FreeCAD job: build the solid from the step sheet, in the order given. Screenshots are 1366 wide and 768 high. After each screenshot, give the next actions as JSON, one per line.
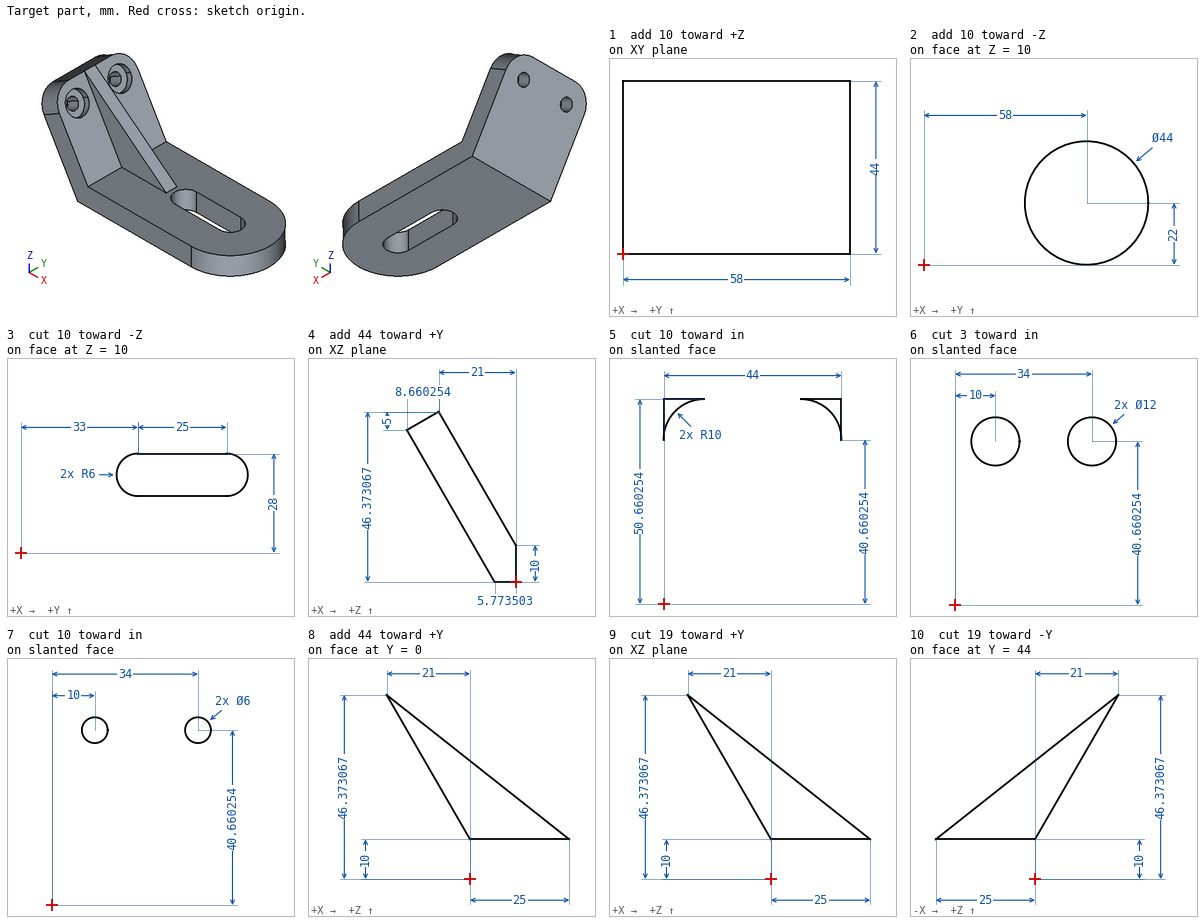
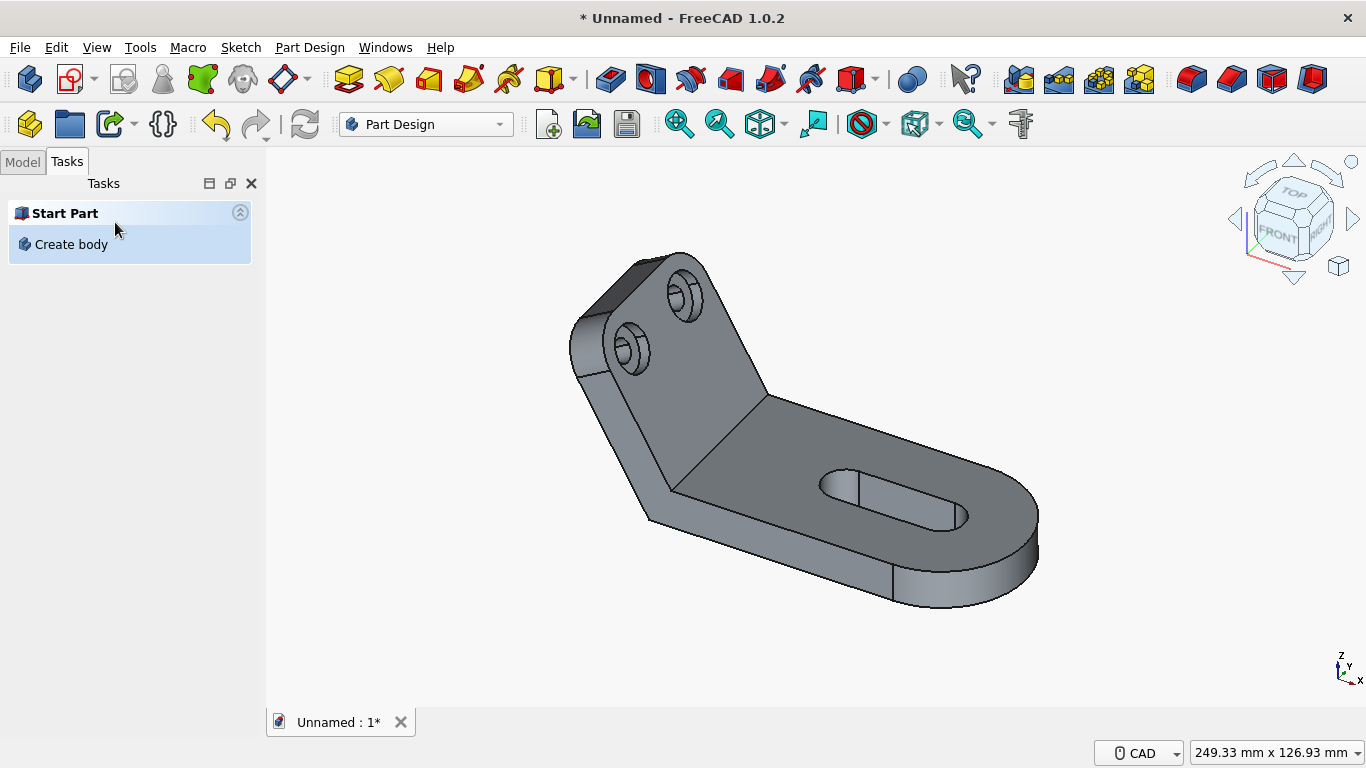
{"action": "left_click", "coordinate": [645, 469]}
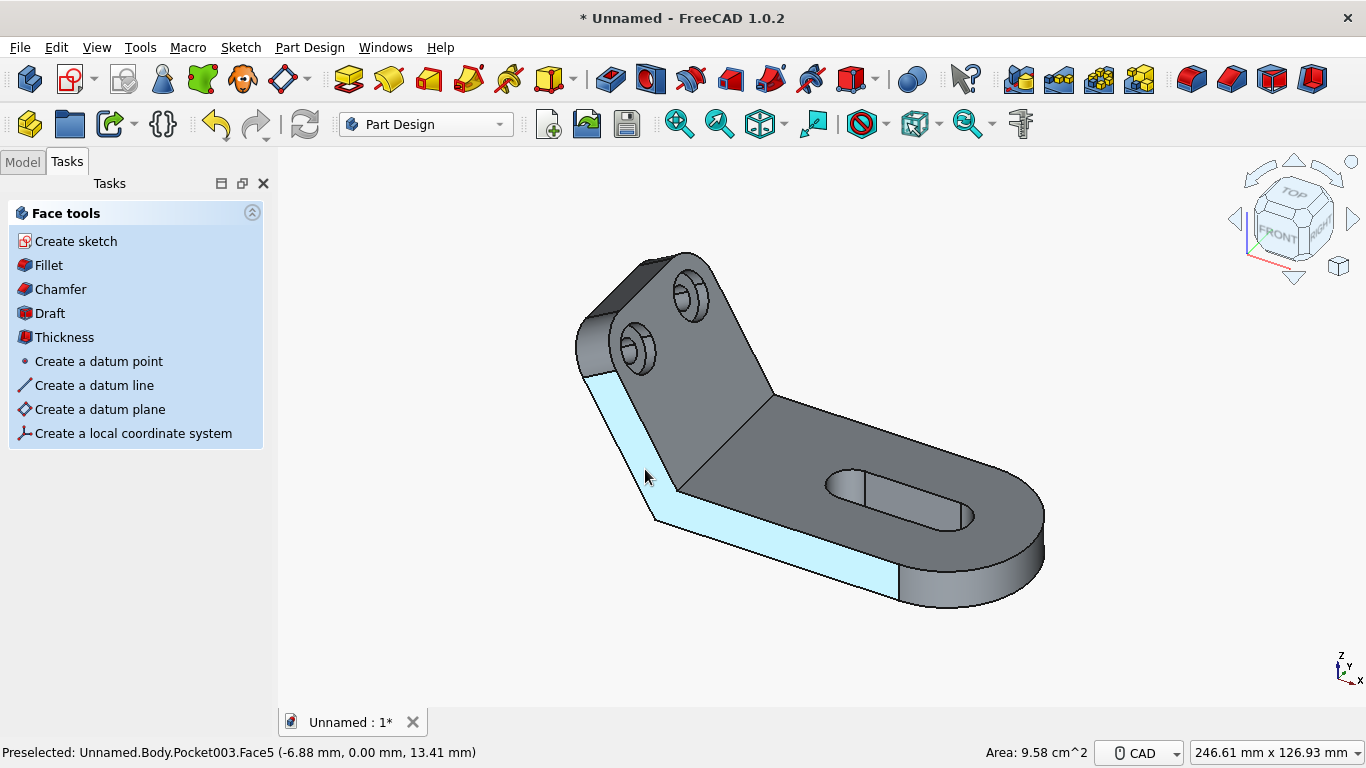
{"action": "left_click", "coordinate": [70, 80]}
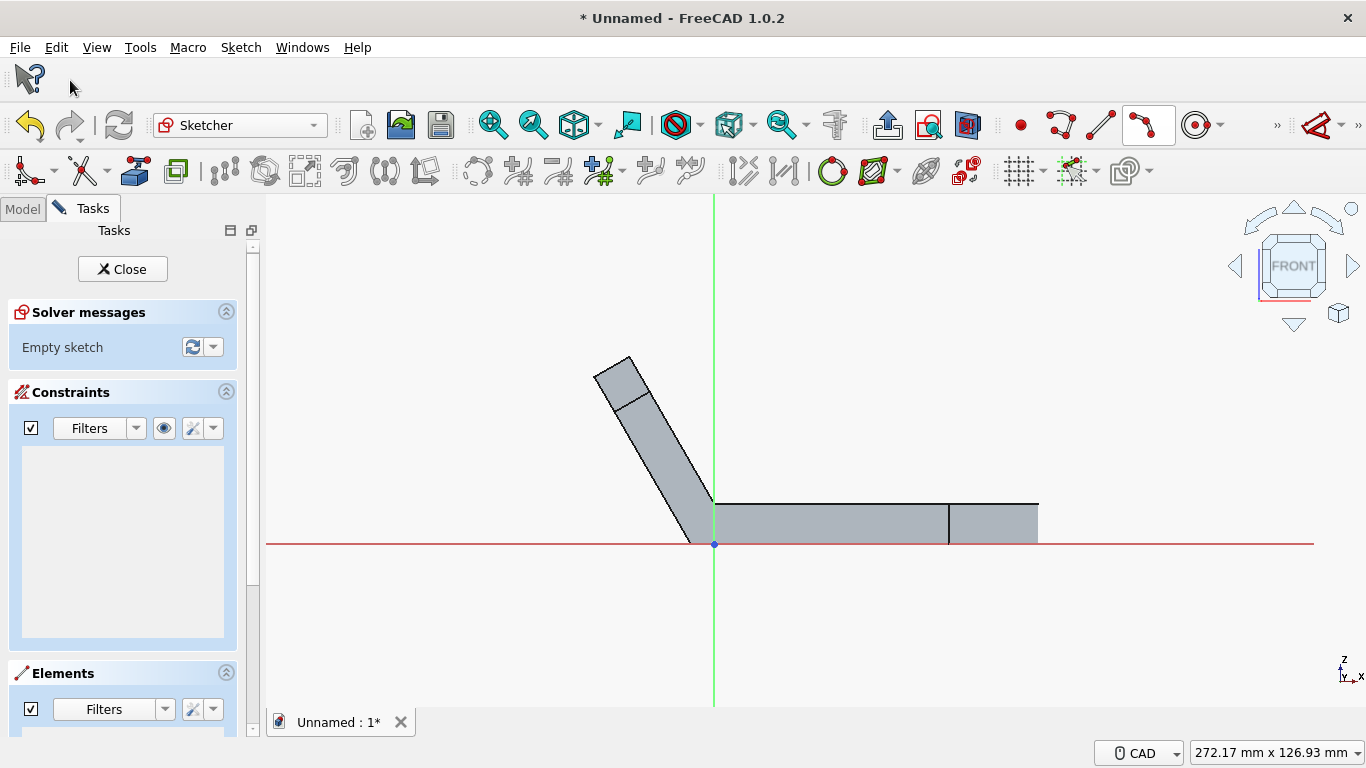
{"action": "scroll", "coordinate": [692, 451], "scroll_direction": "up", "scroll_amount": 3}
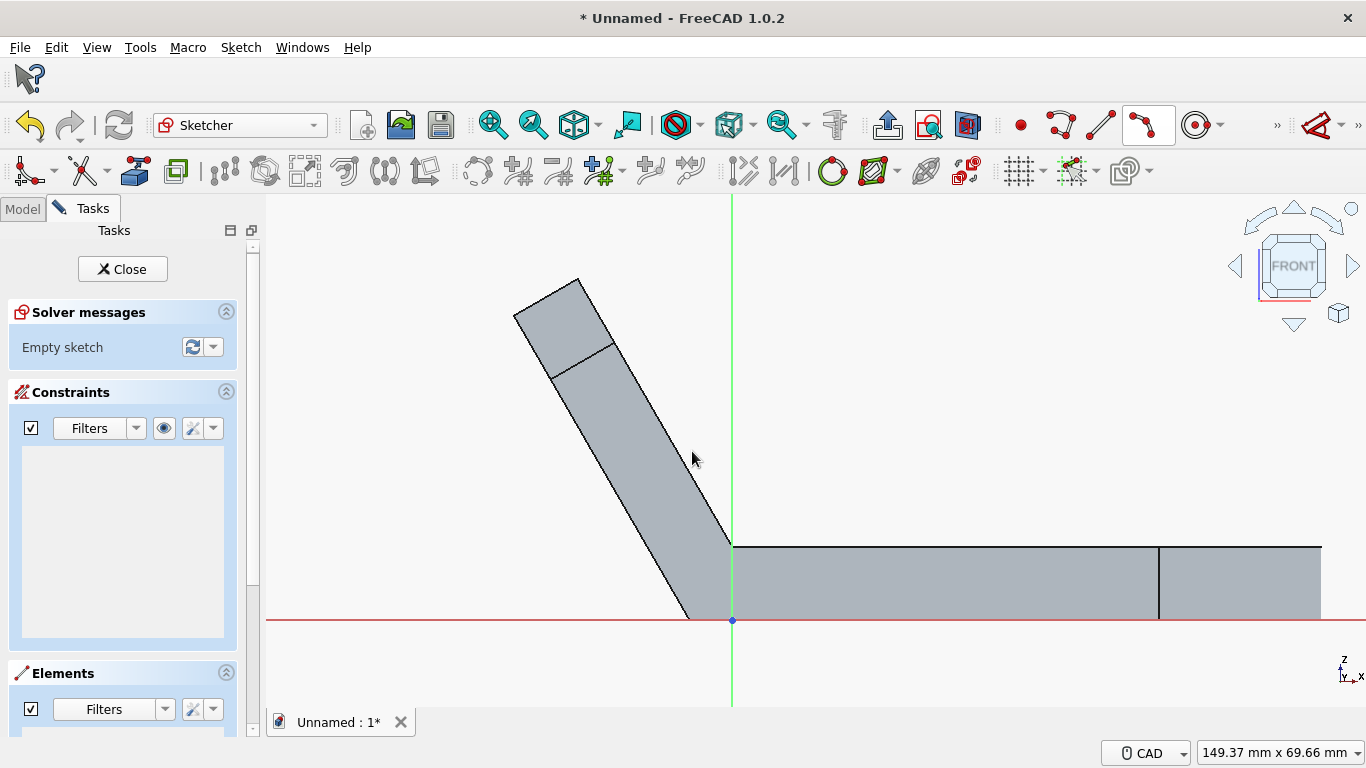
{"action": "left_click", "coordinate": [1062, 126]}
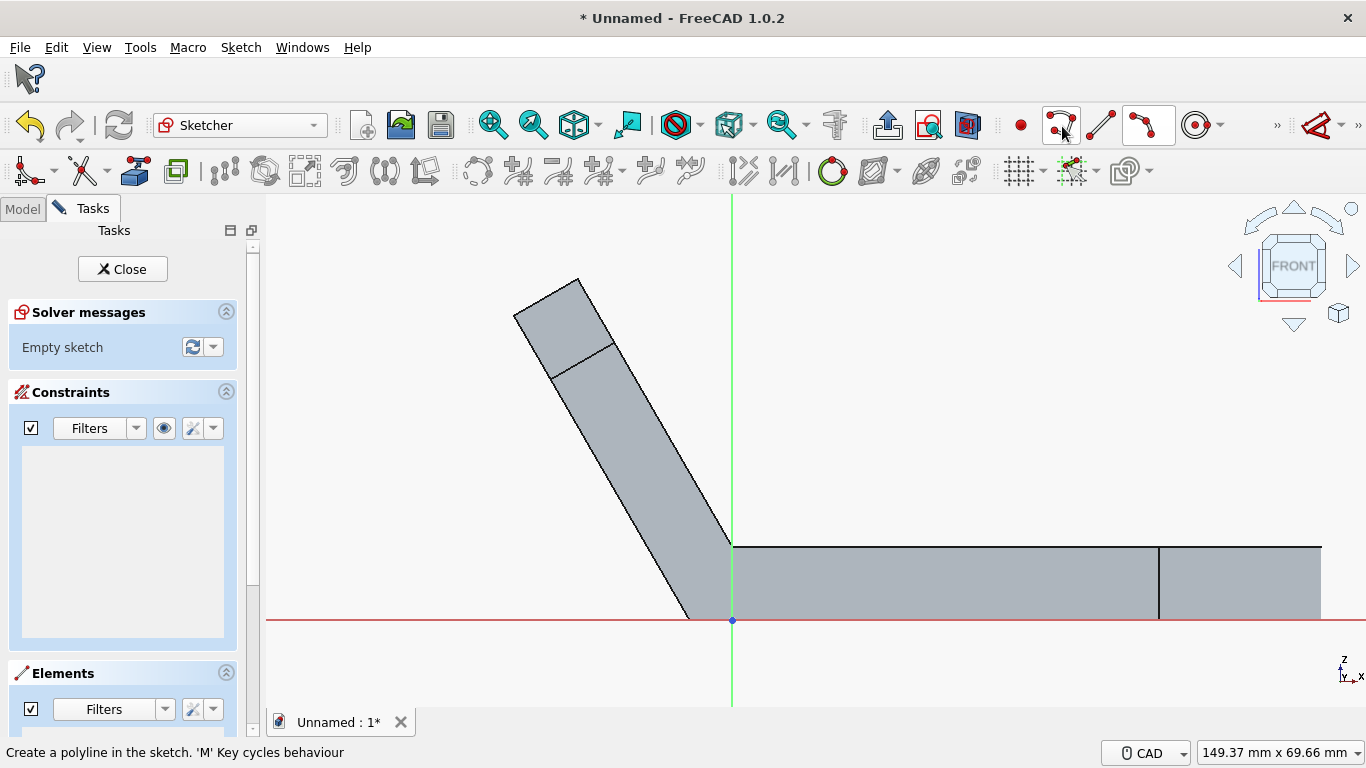
{"action": "left_click", "coordinate": [732, 547]}
{"action": "left_click", "coordinate": [916, 547]}
{"action": "left_click", "coordinate": [578, 279]}
{"action": "left_click", "coordinate": [732, 548]}
{"action": "key", "text": "Escape"}
{"action": "key", "text": "Escape"}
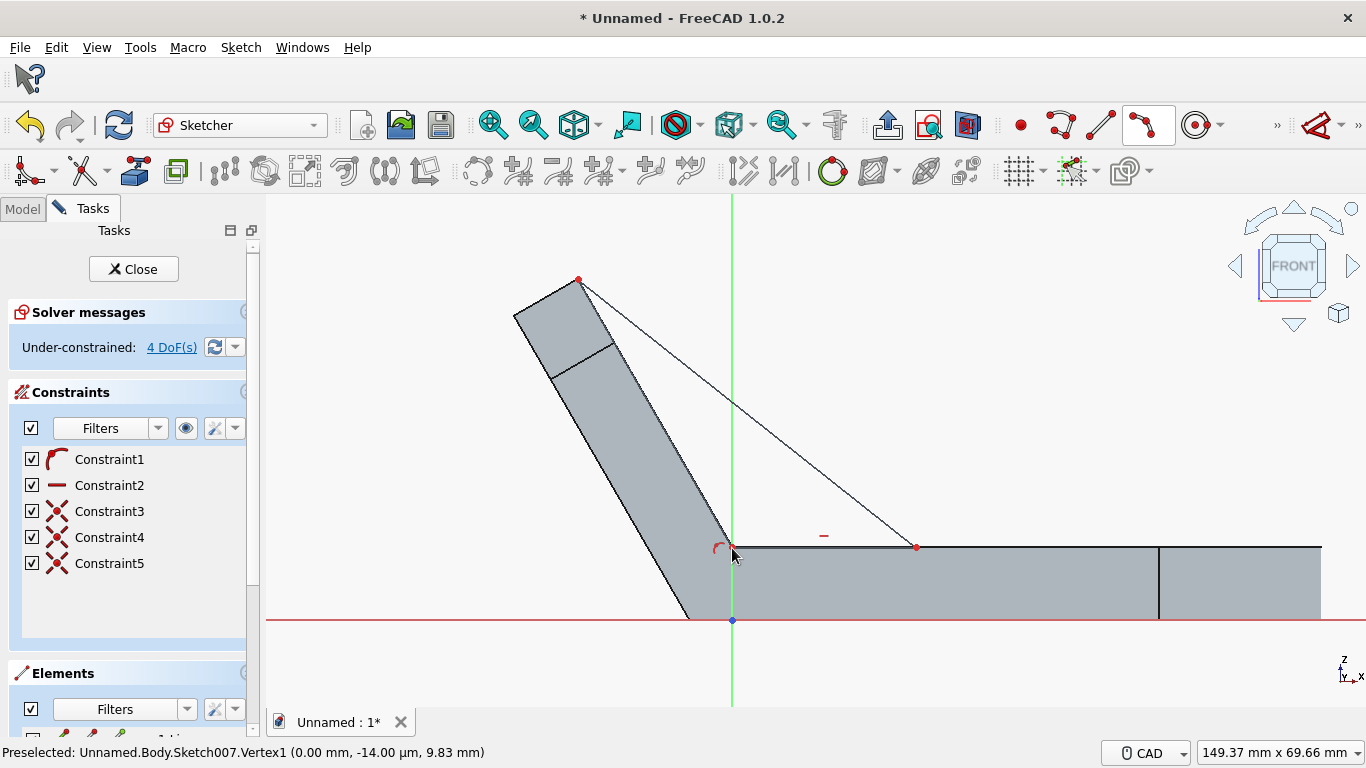
{"action": "left_click", "coordinate": [1316, 126]}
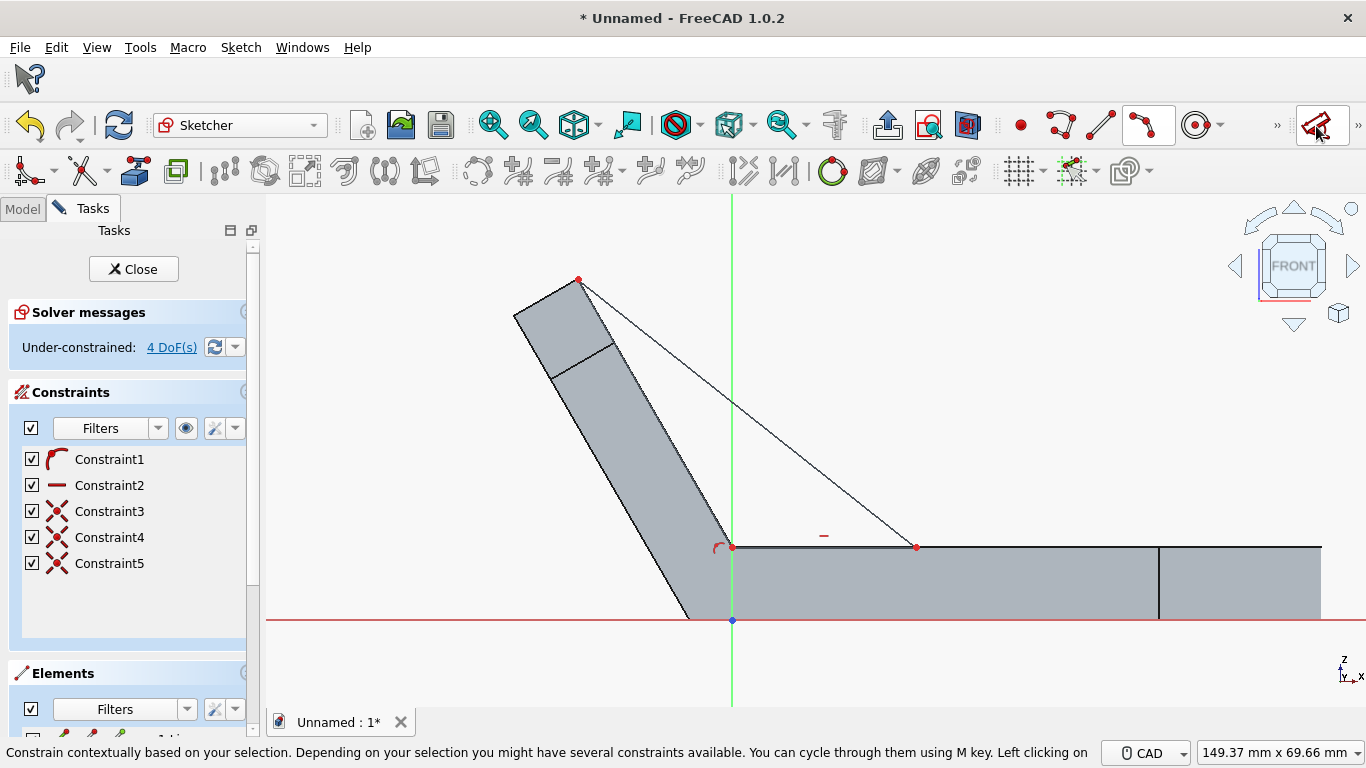
{"action": "left_click", "coordinate": [787, 548]}
{"action": "left_click", "coordinate": [824, 582]}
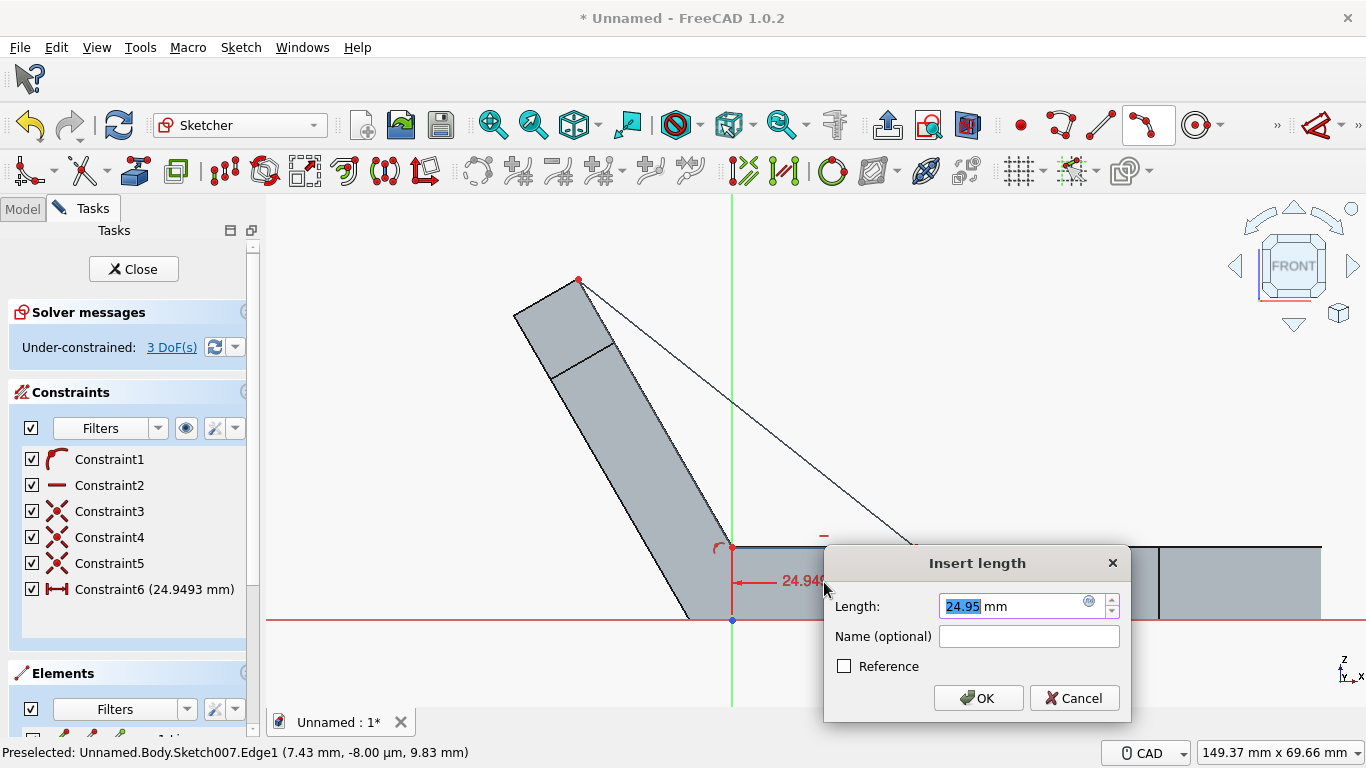
{"action": "type", "text": "25"}
{"action": "key", "text": "Return"}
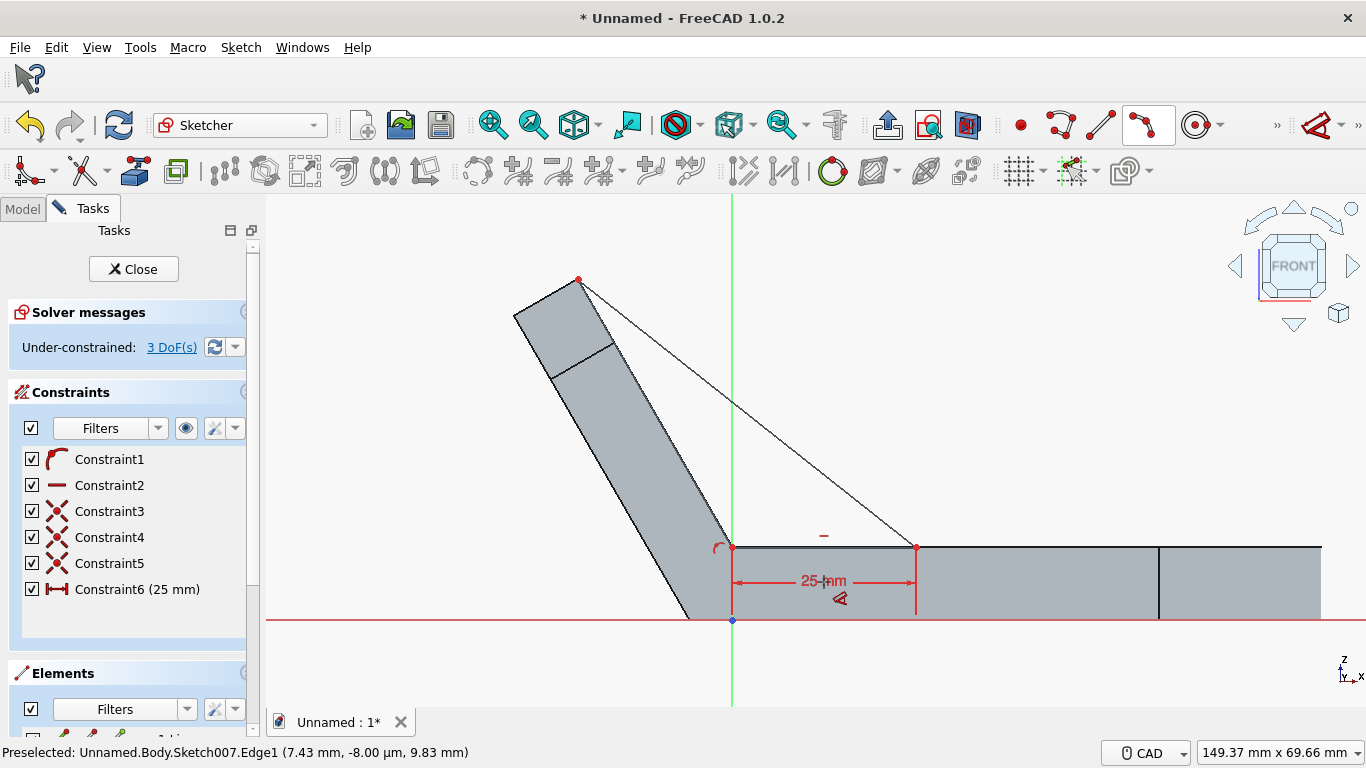
{"action": "left_click", "coordinate": [732, 548]}
{"action": "left_click", "coordinate": [698, 584]}